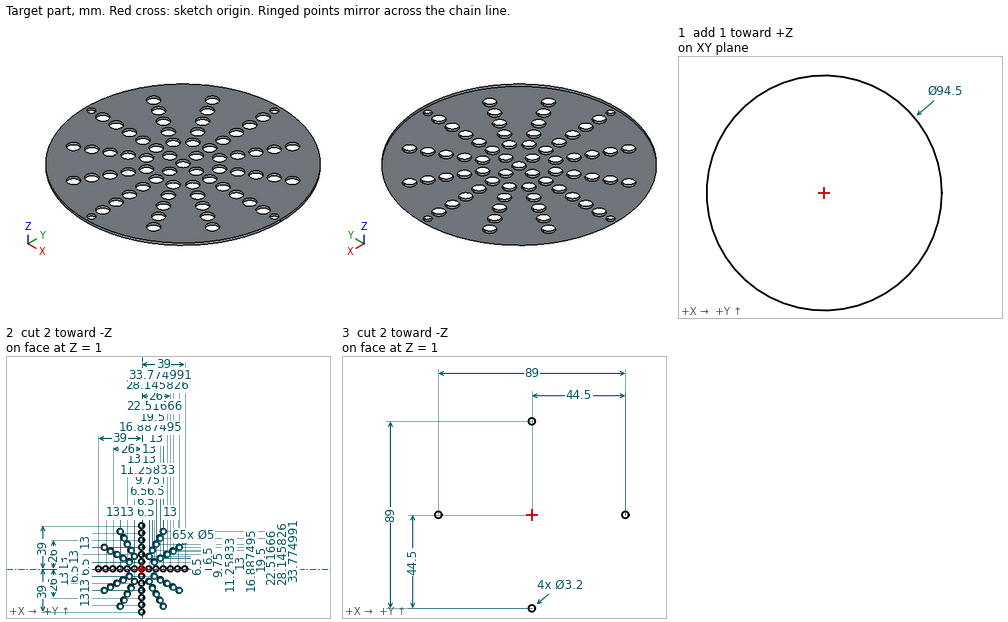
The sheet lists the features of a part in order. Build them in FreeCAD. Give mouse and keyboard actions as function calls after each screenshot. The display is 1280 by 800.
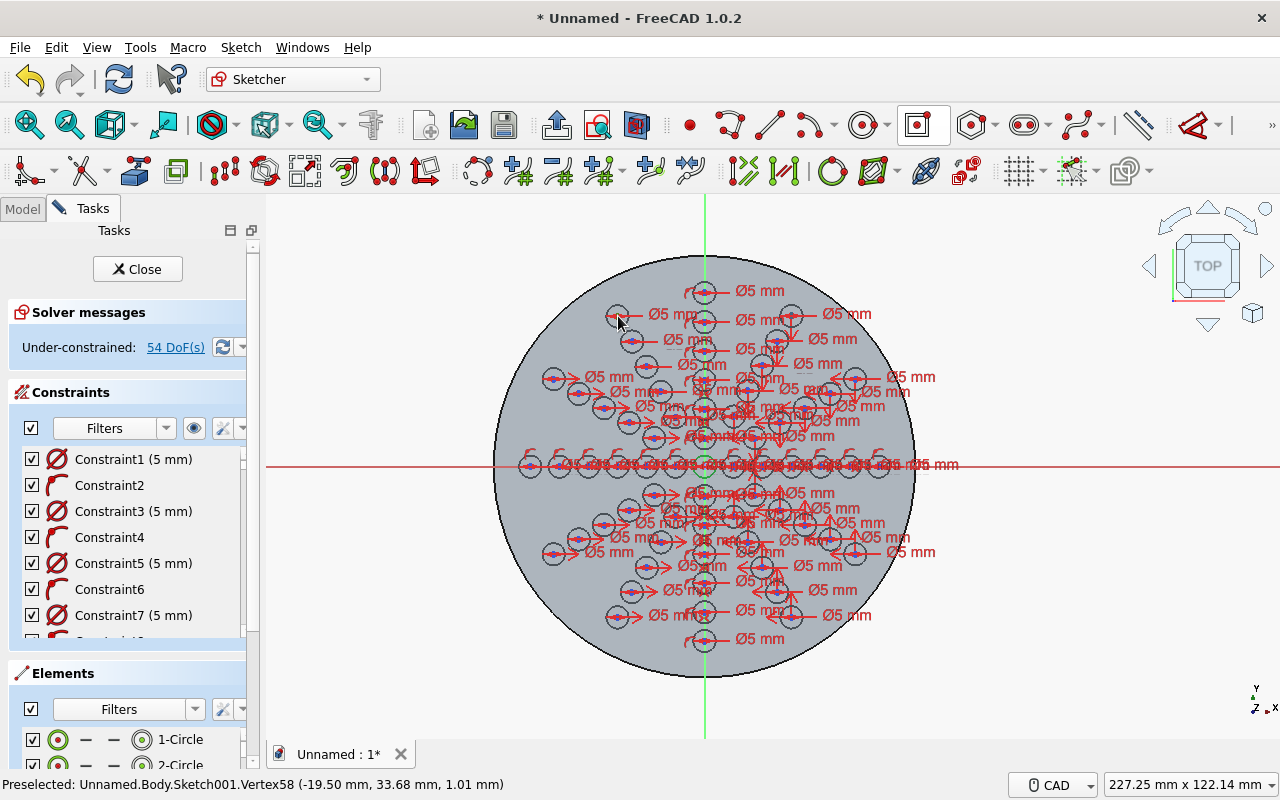
click(705, 257)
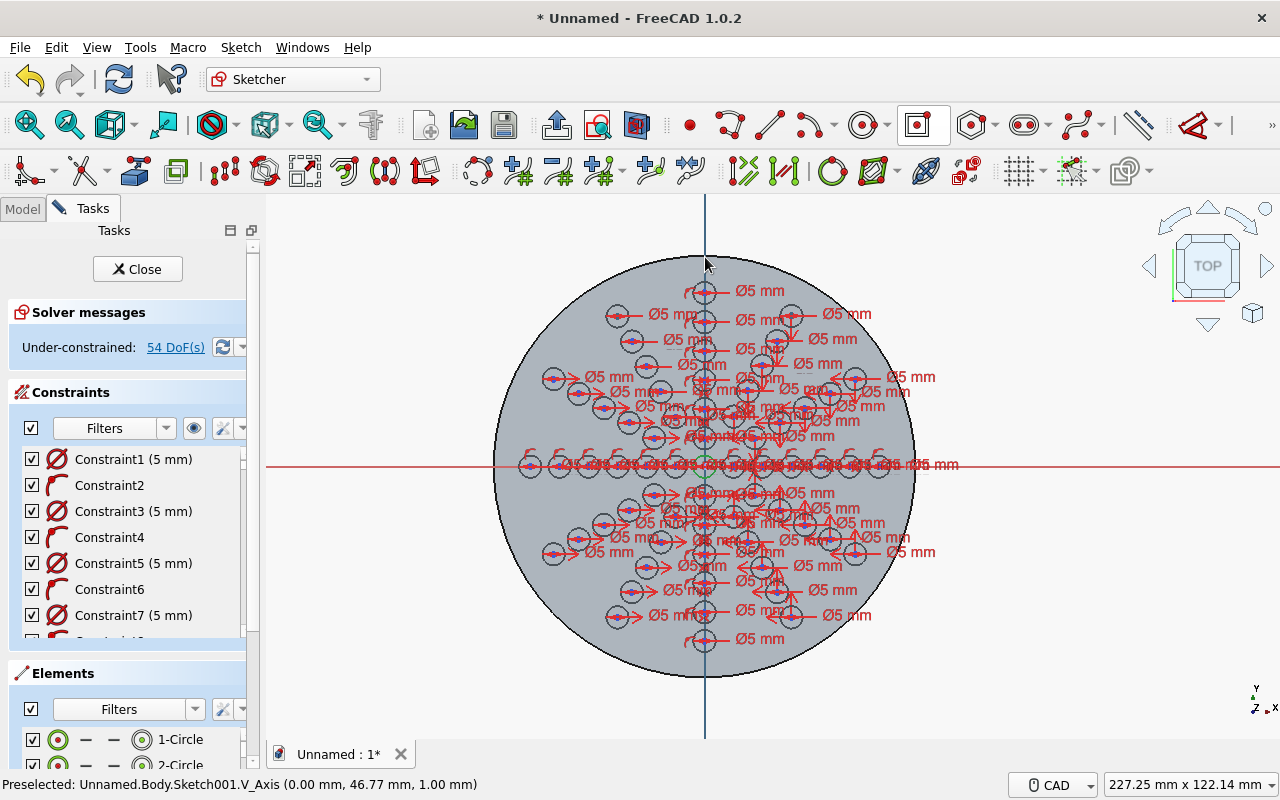
key(s)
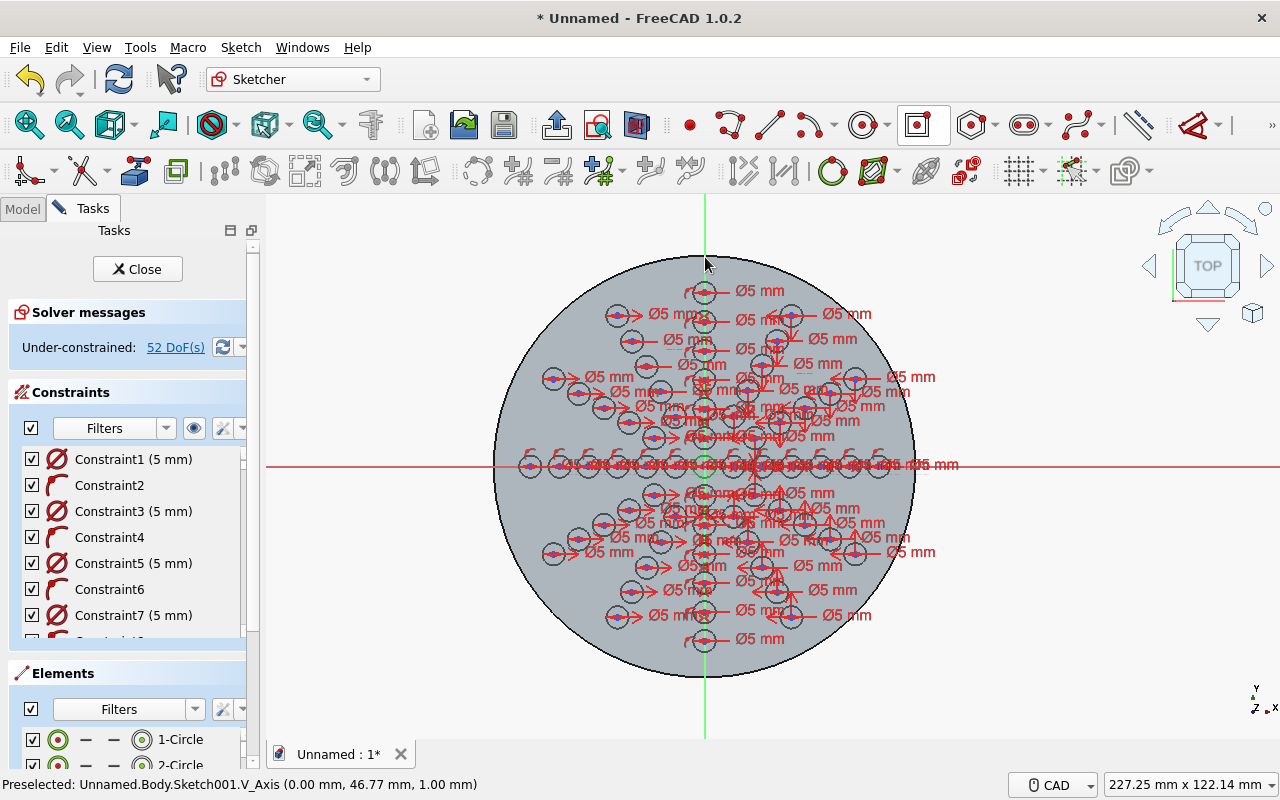
click(777, 341)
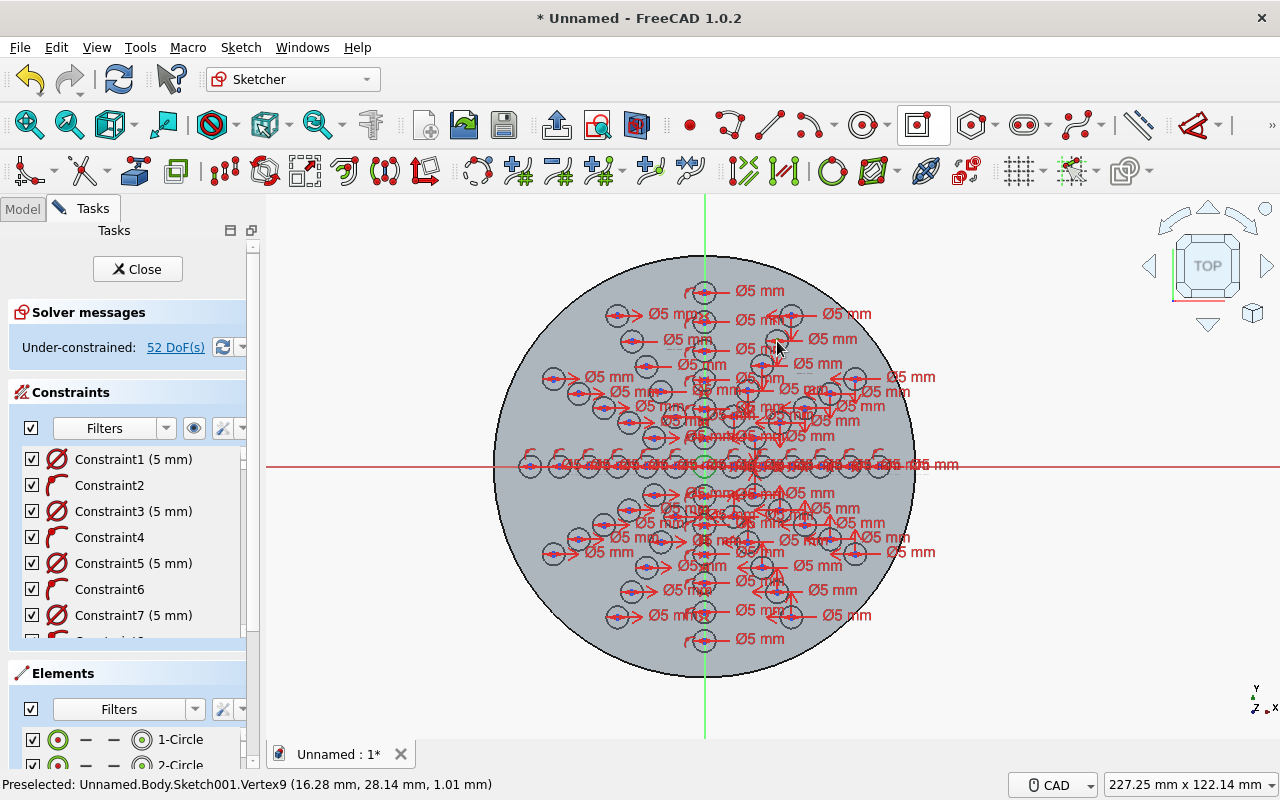
click(632, 342)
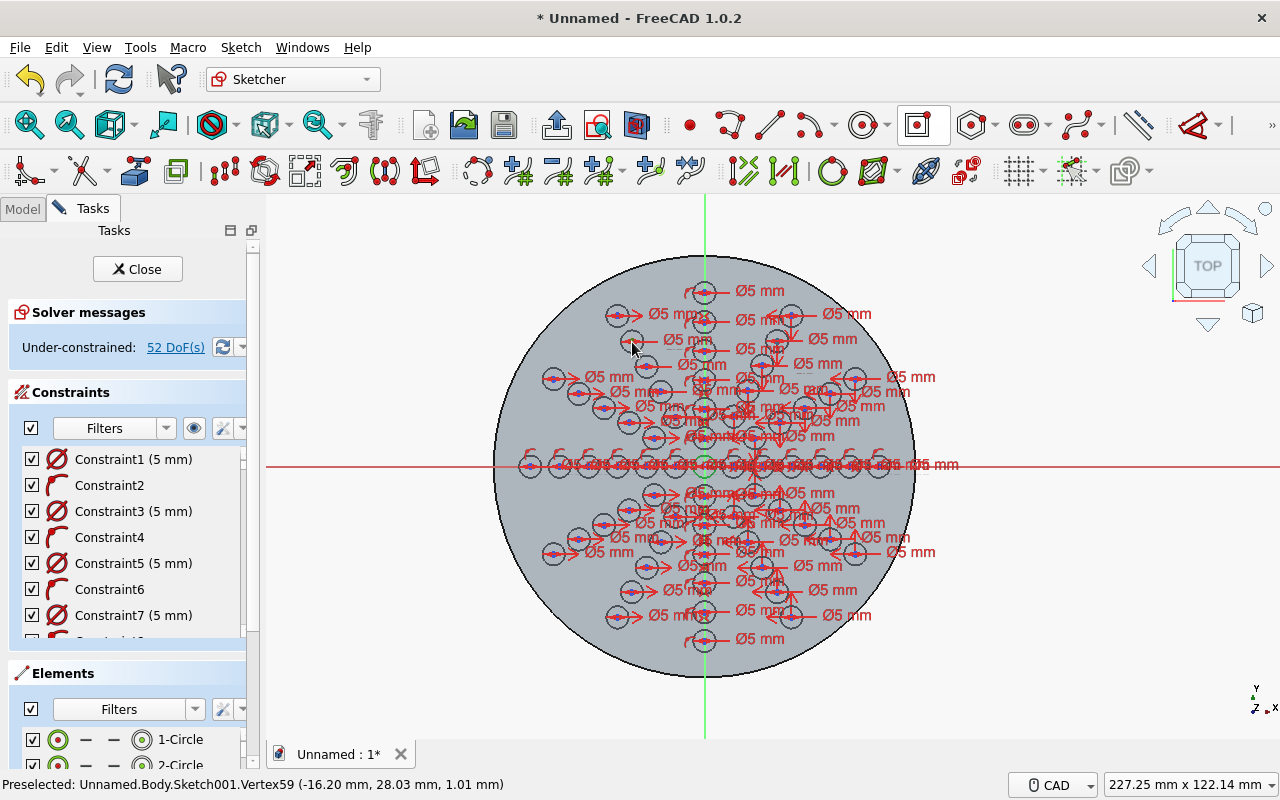
click(705, 257)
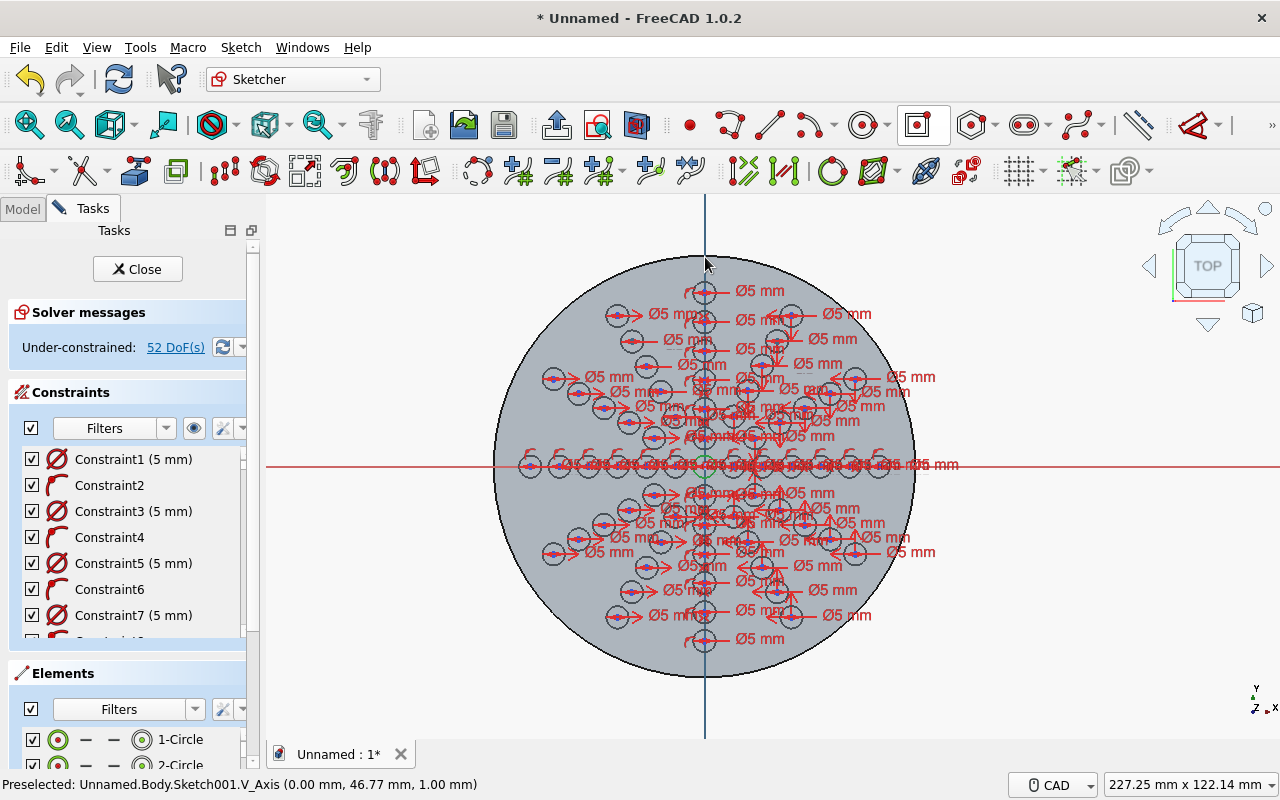
key(s)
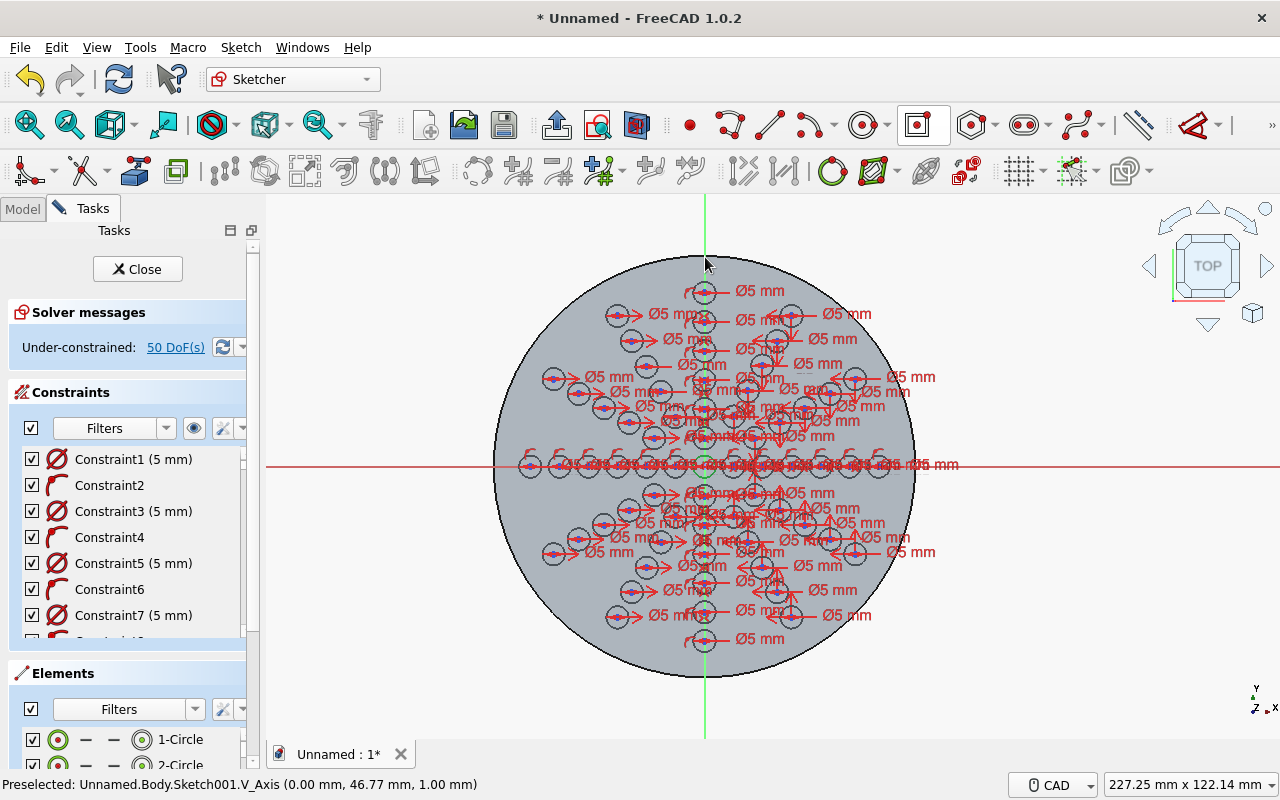
click(762, 366)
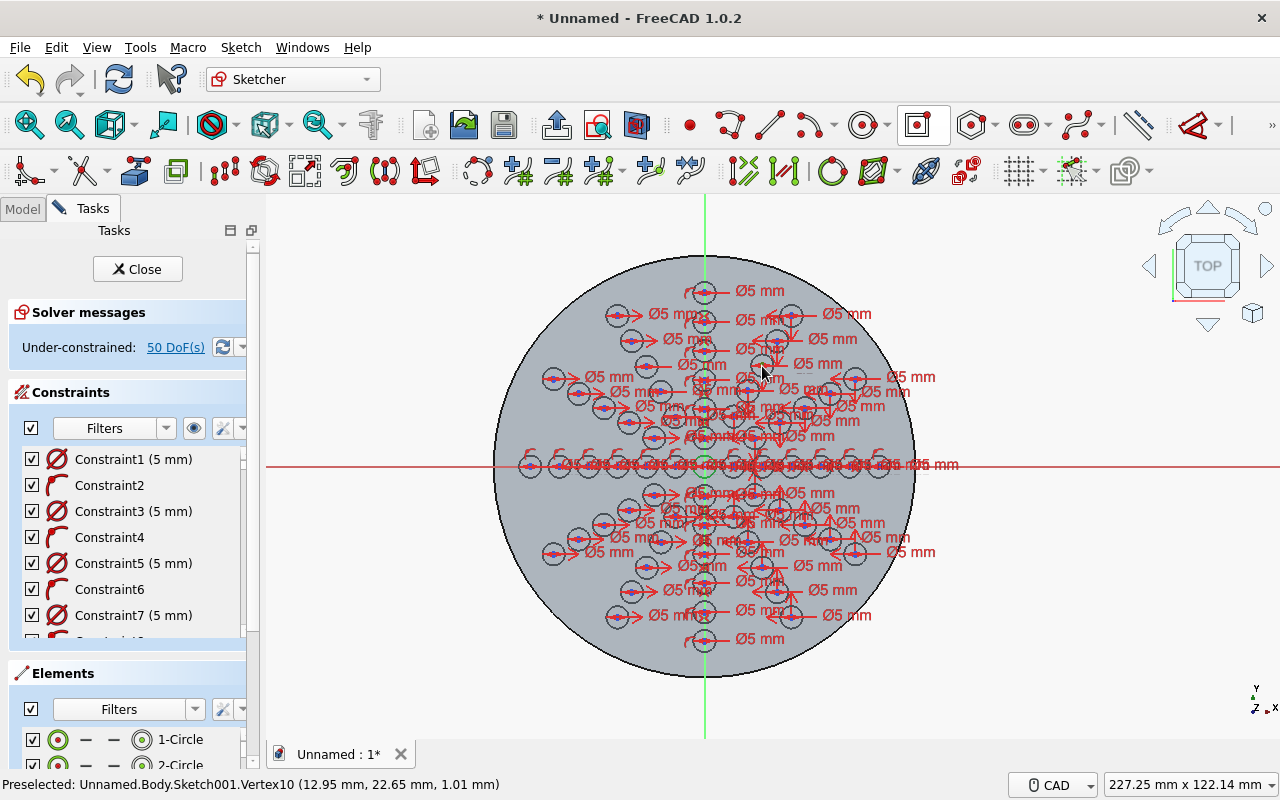
click(647, 367)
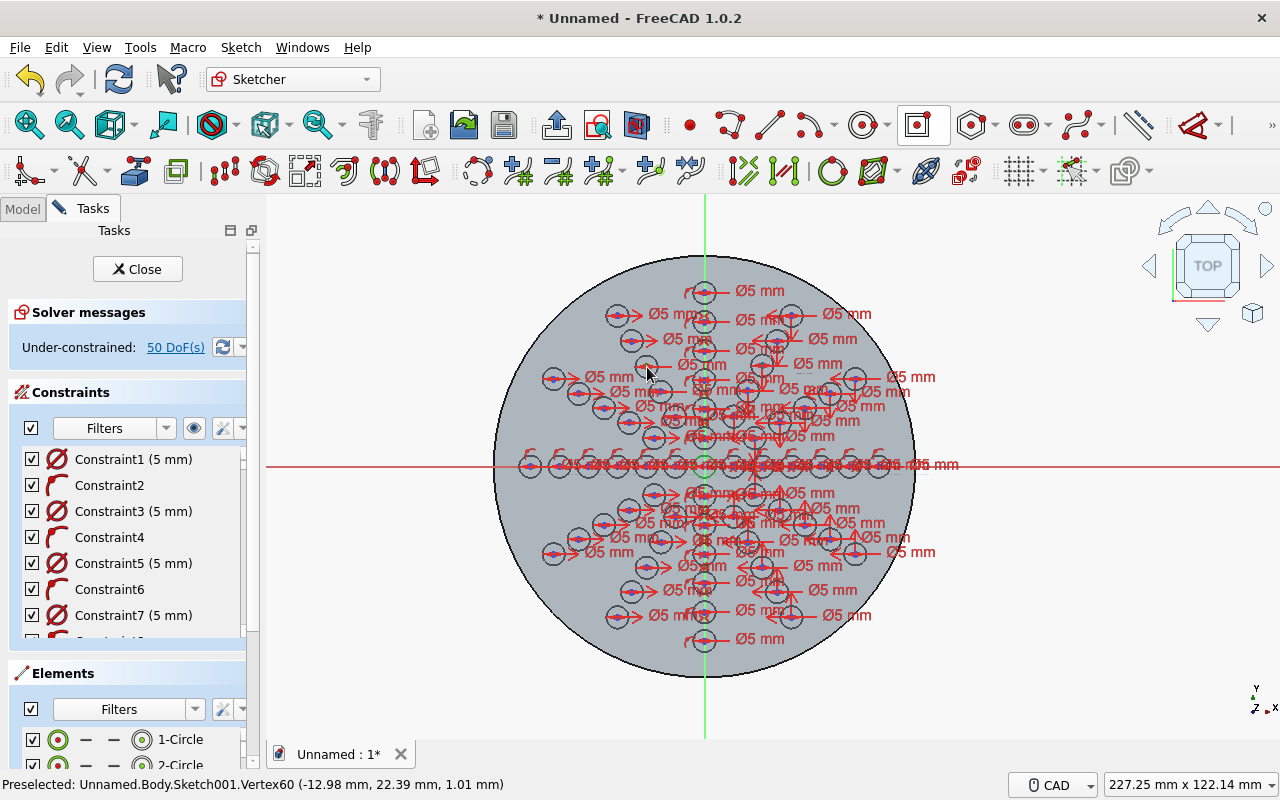
click(705, 257)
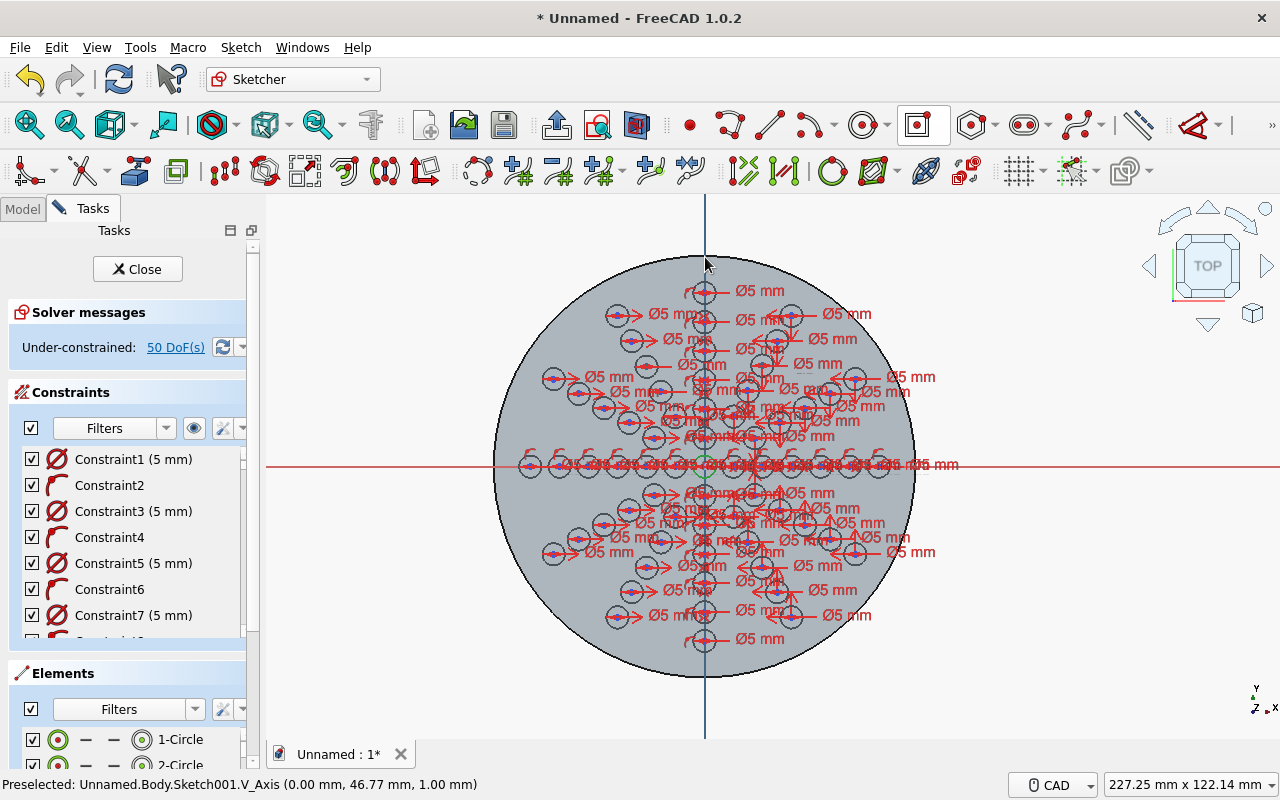
key(s)